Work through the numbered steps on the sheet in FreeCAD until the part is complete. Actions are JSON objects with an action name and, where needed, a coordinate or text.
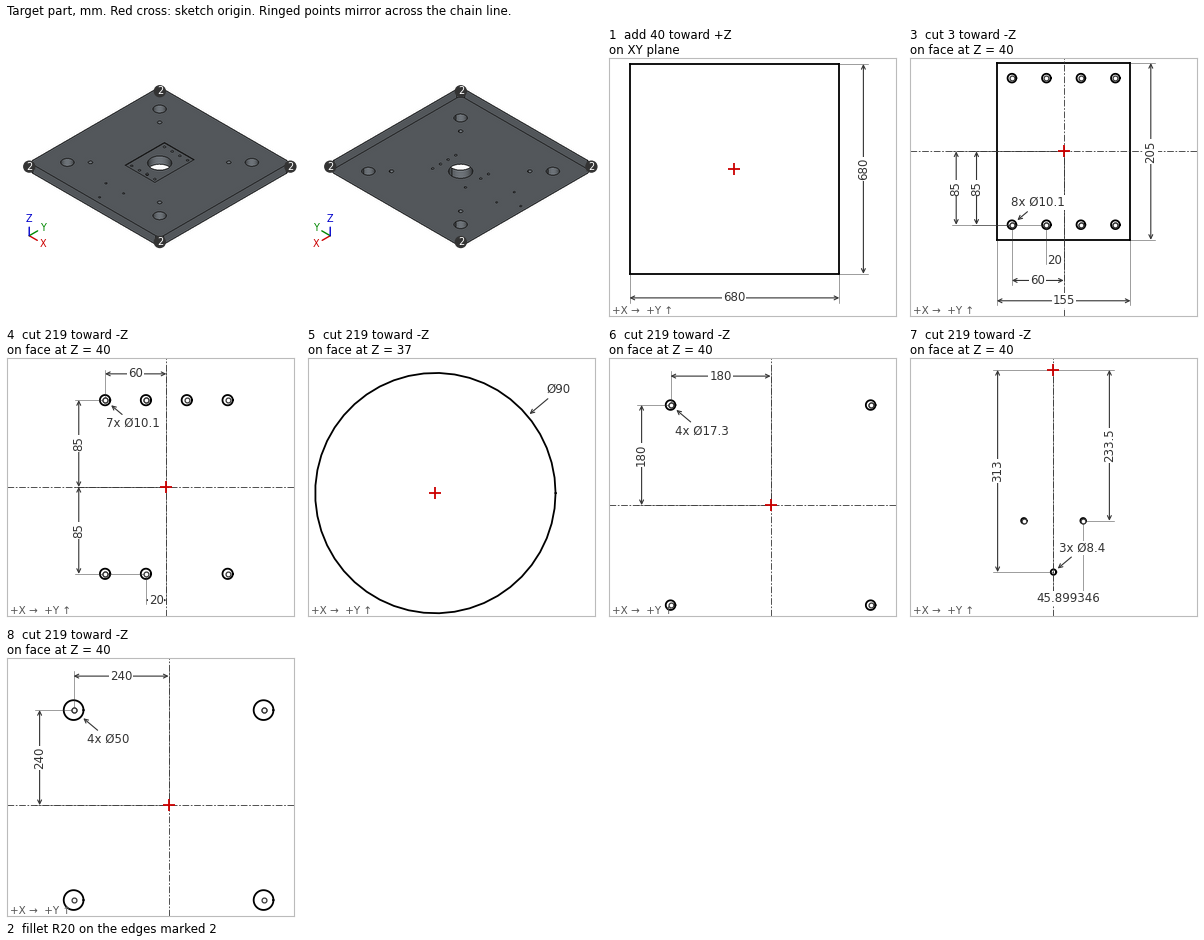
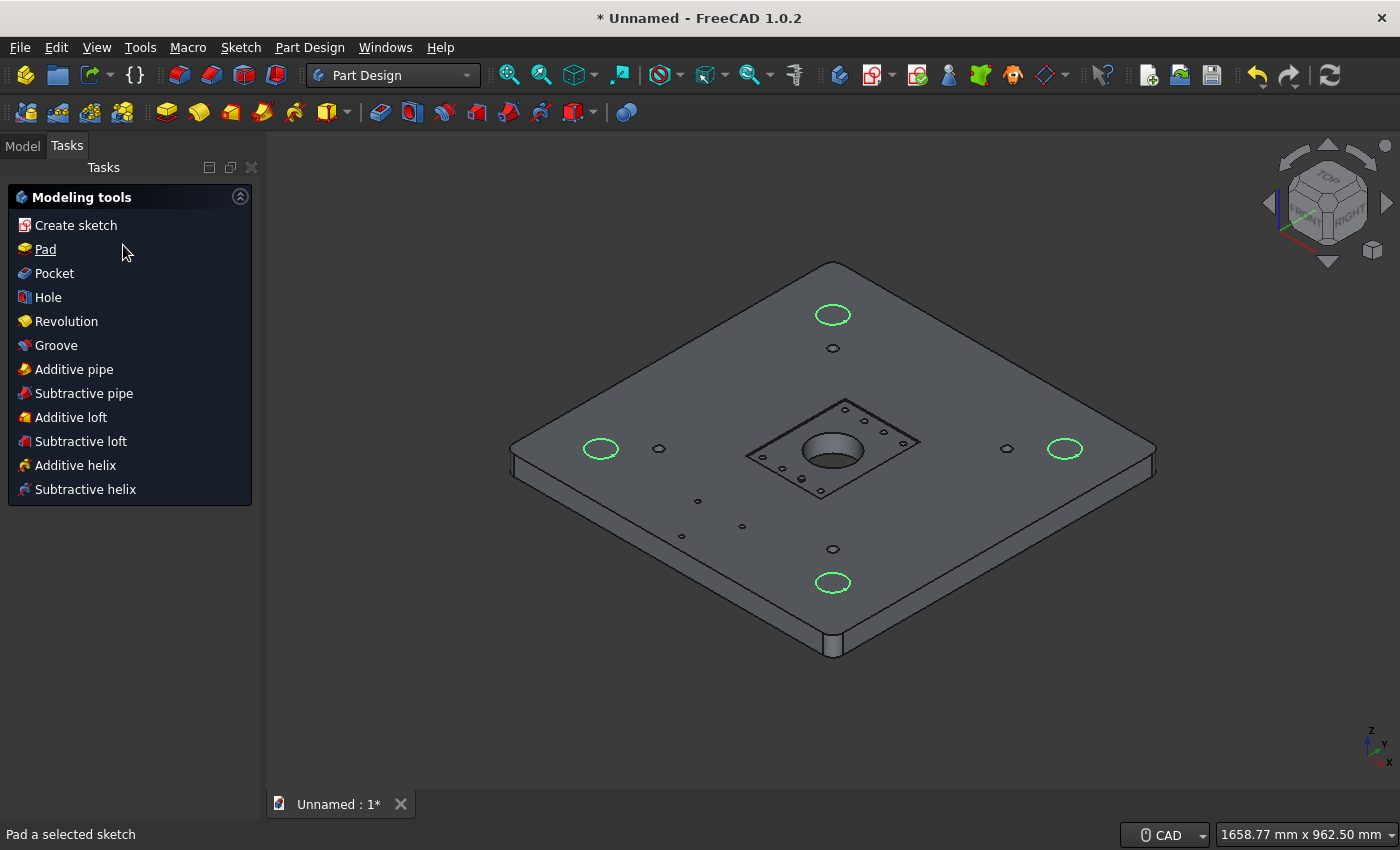
{"action": "left_click", "coordinate": [382, 112]}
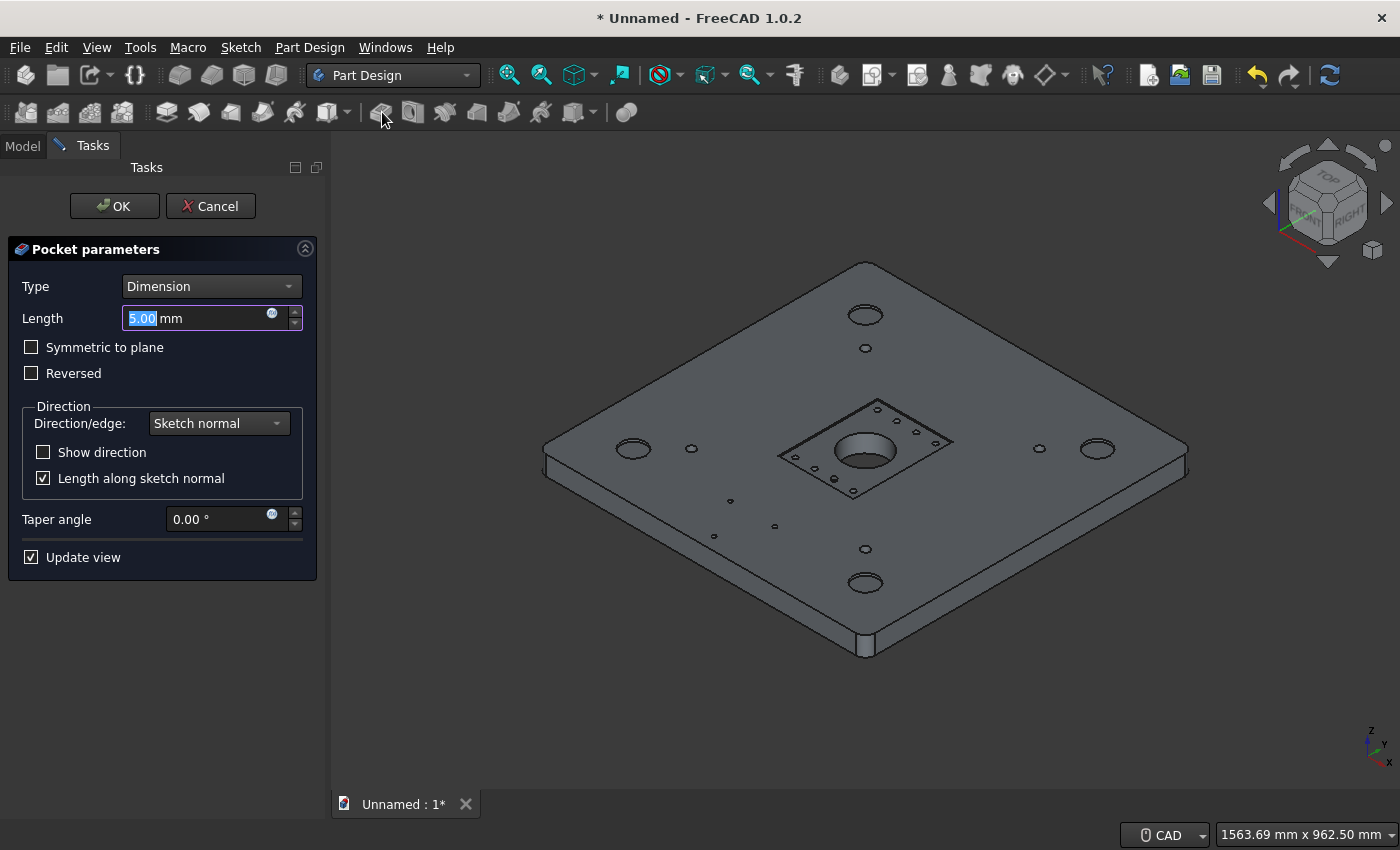
{"action": "type", "text": "219"}
{"action": "key", "text": "Tab"}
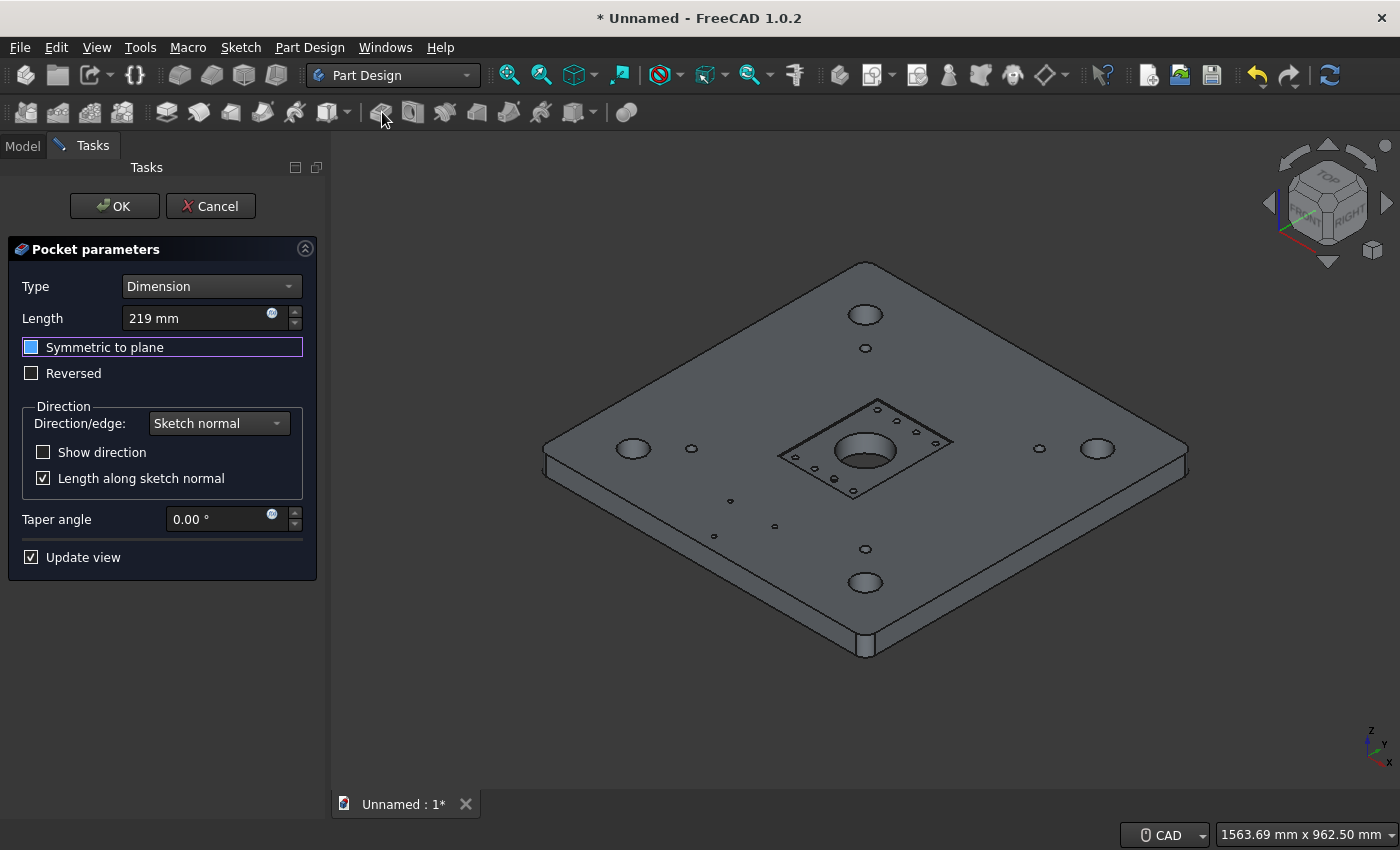
{"action": "left_click", "coordinate": [115, 206]}